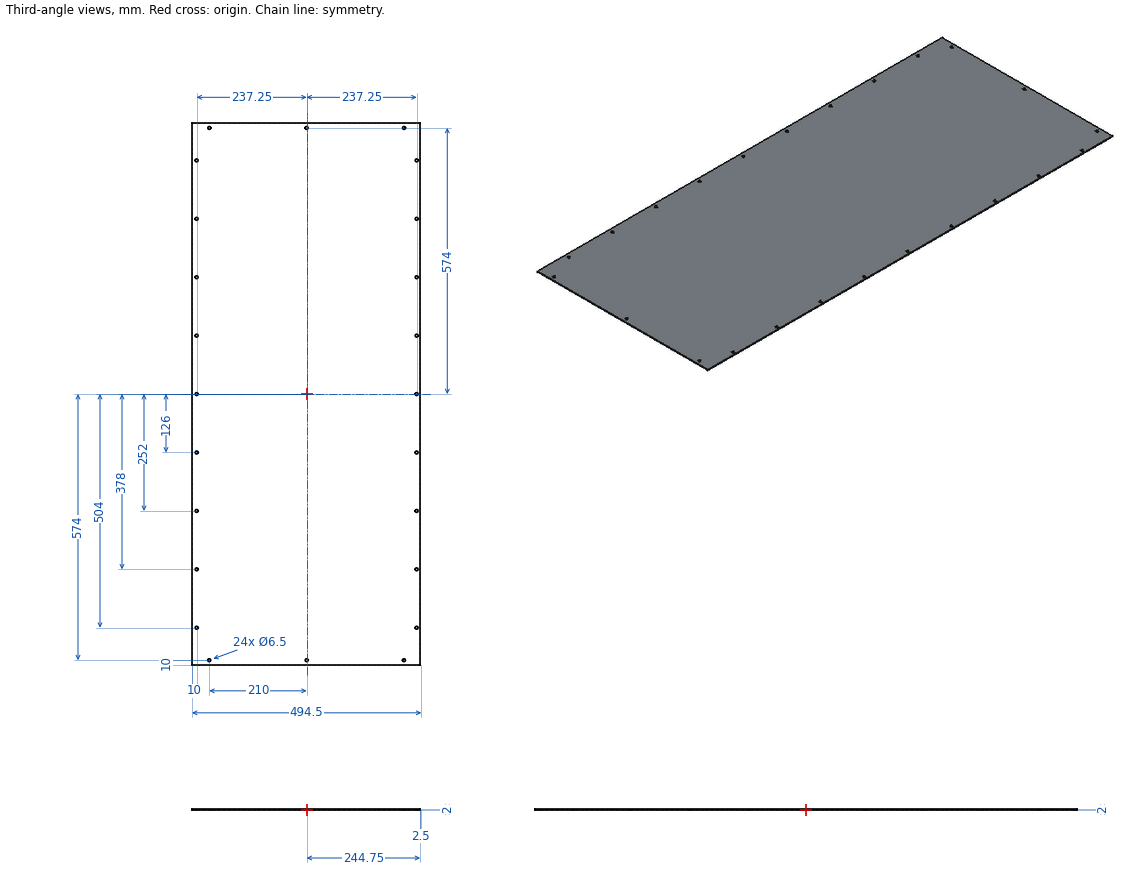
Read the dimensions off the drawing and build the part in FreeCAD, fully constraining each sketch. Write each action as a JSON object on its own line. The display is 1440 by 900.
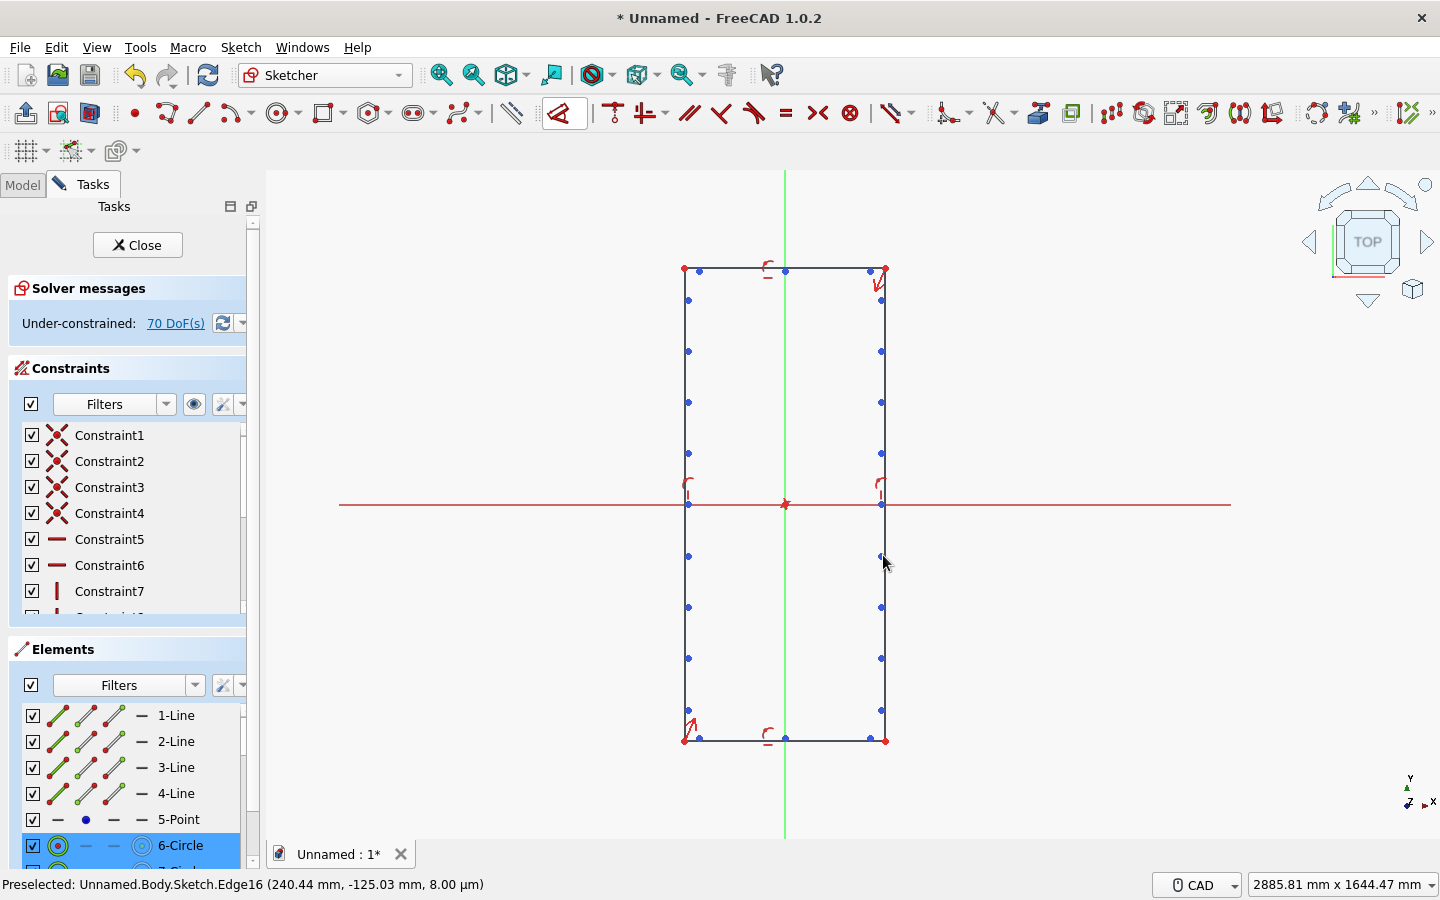
{"action": "scroll", "coordinate": [690, 504], "scroll_direction": "up", "scroll_amount": 14}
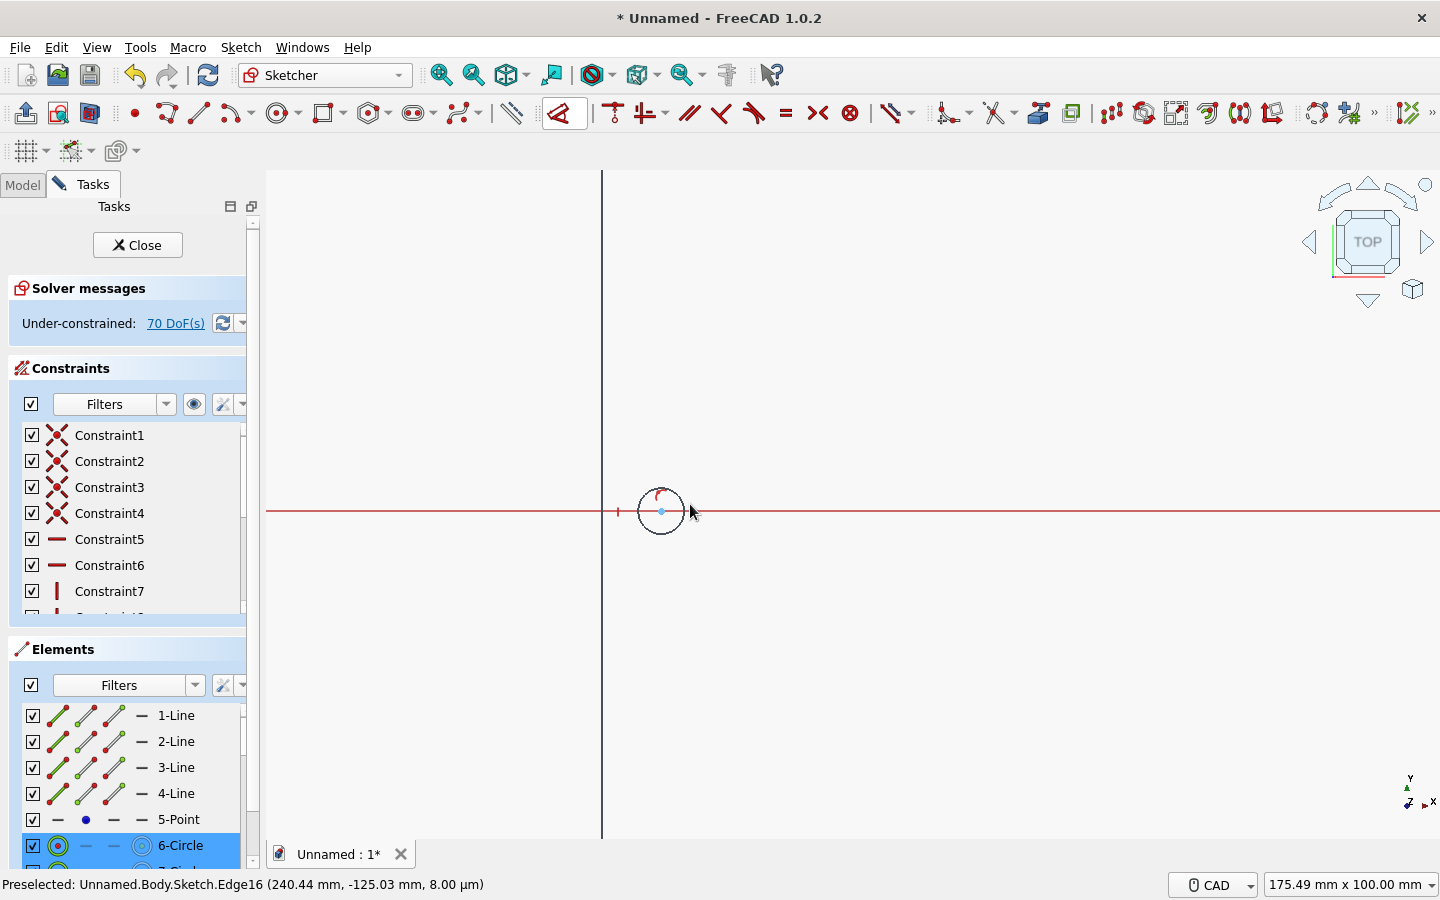
{"action": "left_click", "coordinate": [677, 495]}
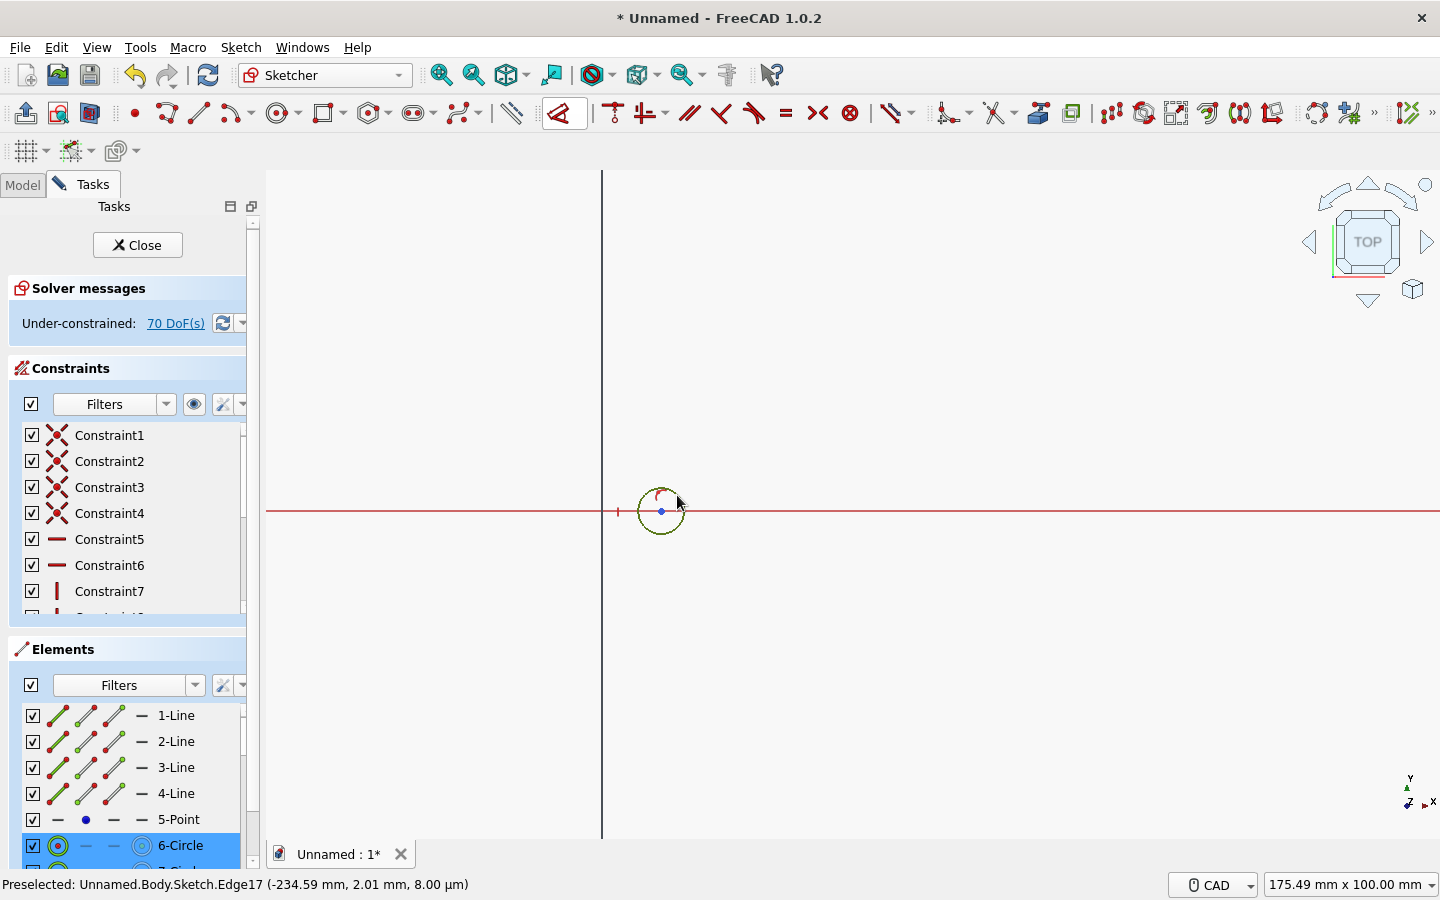
{"action": "scroll", "coordinate": [690, 504], "scroll_direction": "down", "scroll_amount": 14}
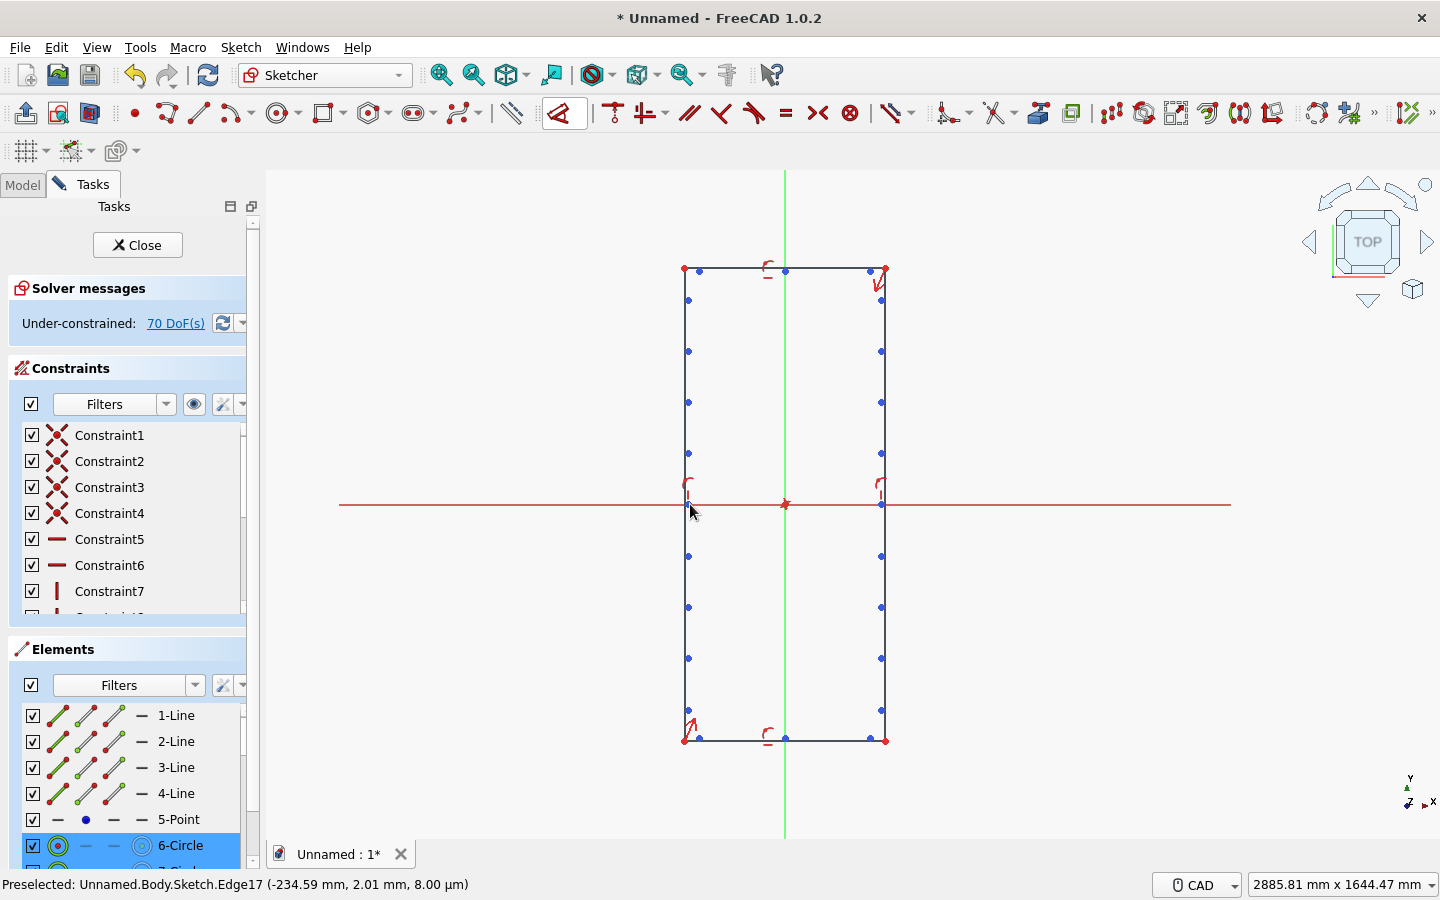
{"action": "scroll", "coordinate": [690, 453], "scroll_direction": "up", "scroll_amount": 12}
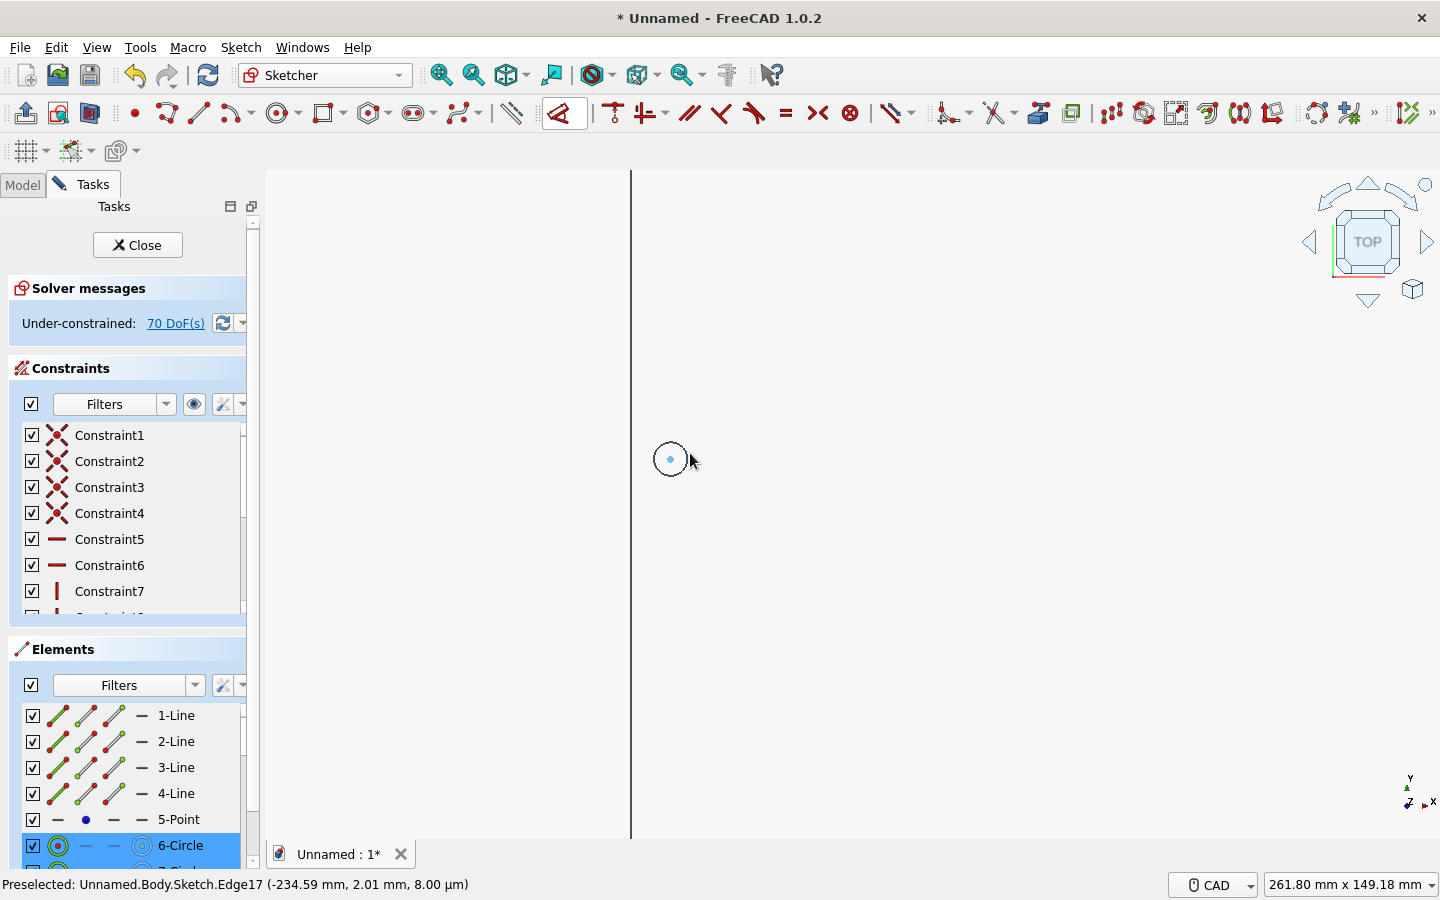
{"action": "left_click", "coordinate": [682, 447]}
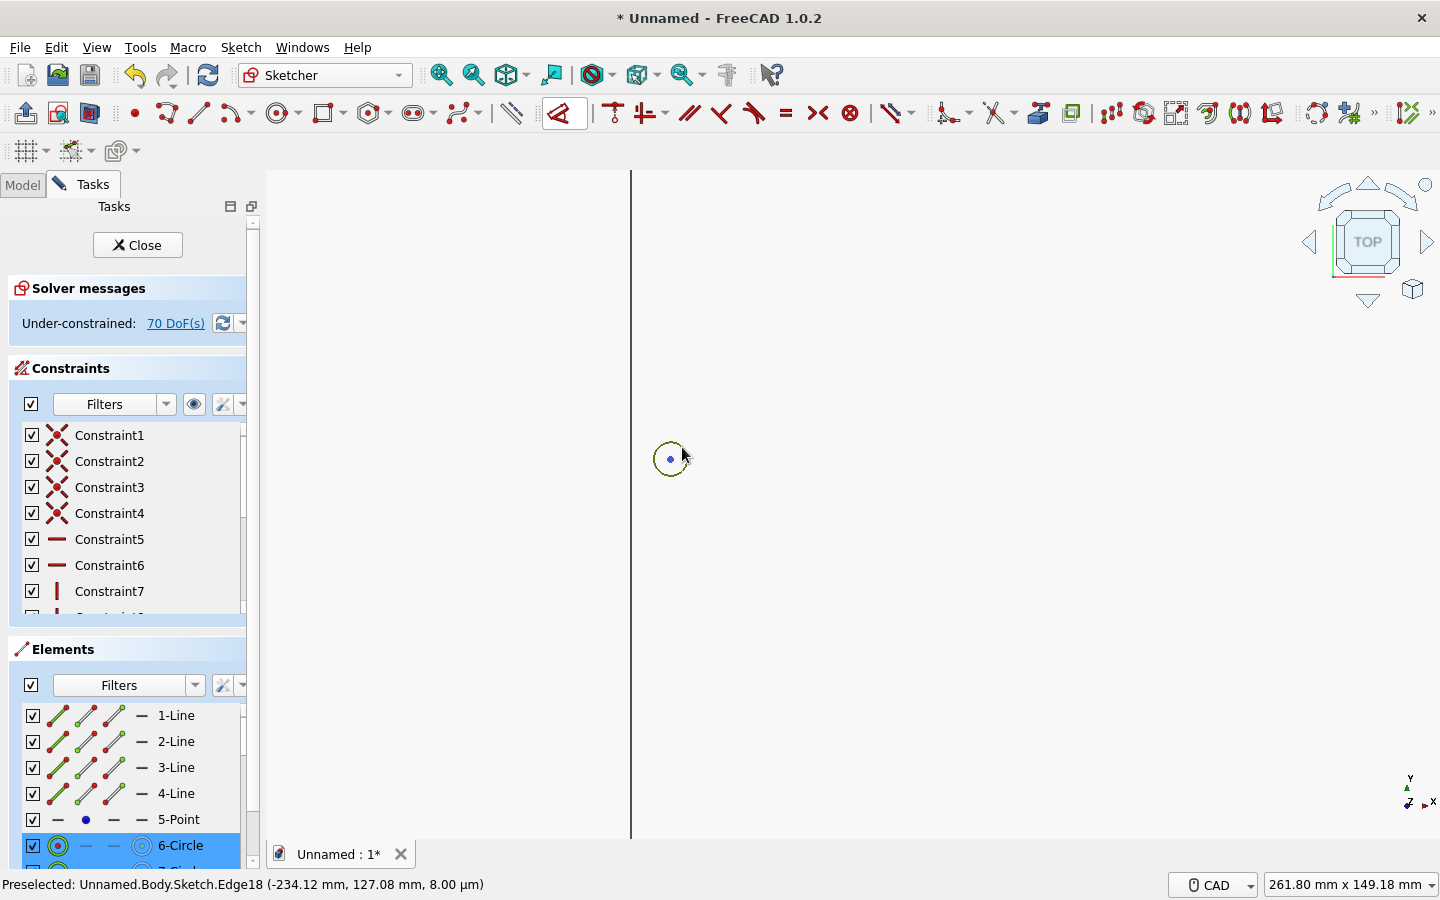
{"action": "scroll", "coordinate": [690, 453], "scroll_direction": "down", "scroll_amount": 12}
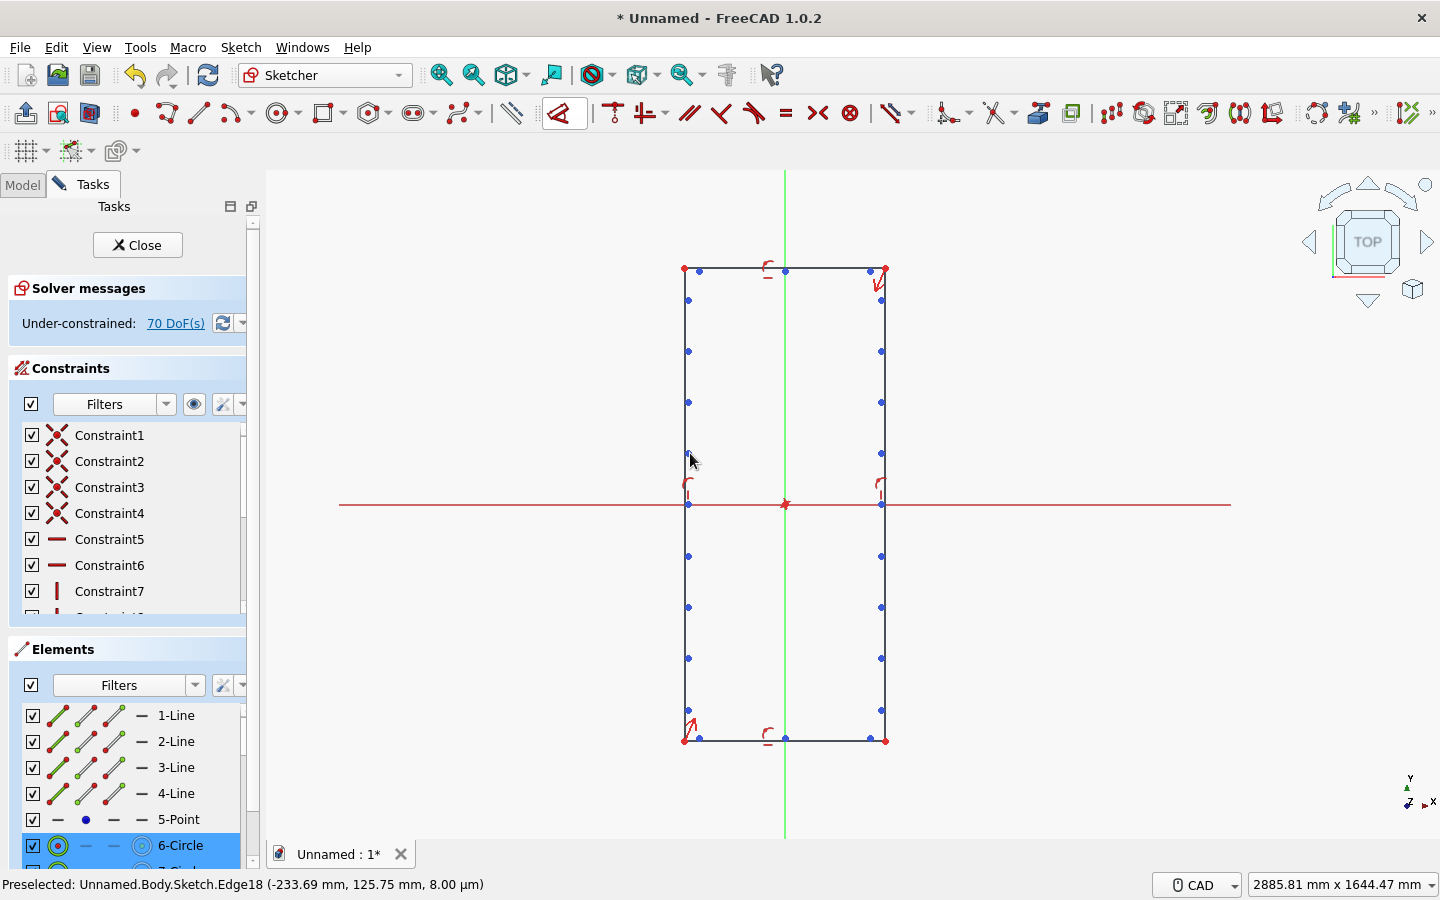
{"action": "scroll", "coordinate": [690, 402], "scroll_direction": "up", "scroll_amount": 12}